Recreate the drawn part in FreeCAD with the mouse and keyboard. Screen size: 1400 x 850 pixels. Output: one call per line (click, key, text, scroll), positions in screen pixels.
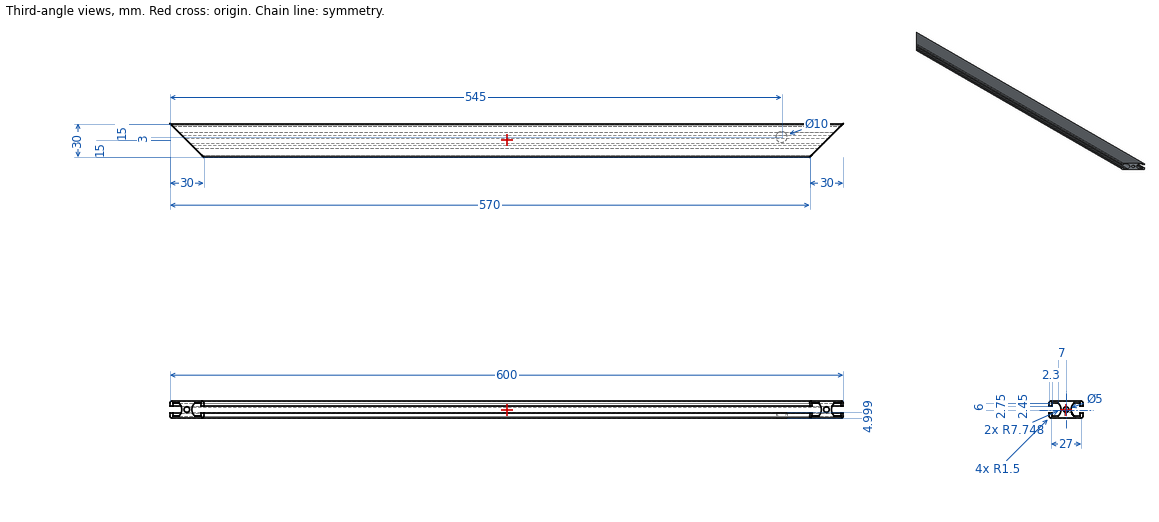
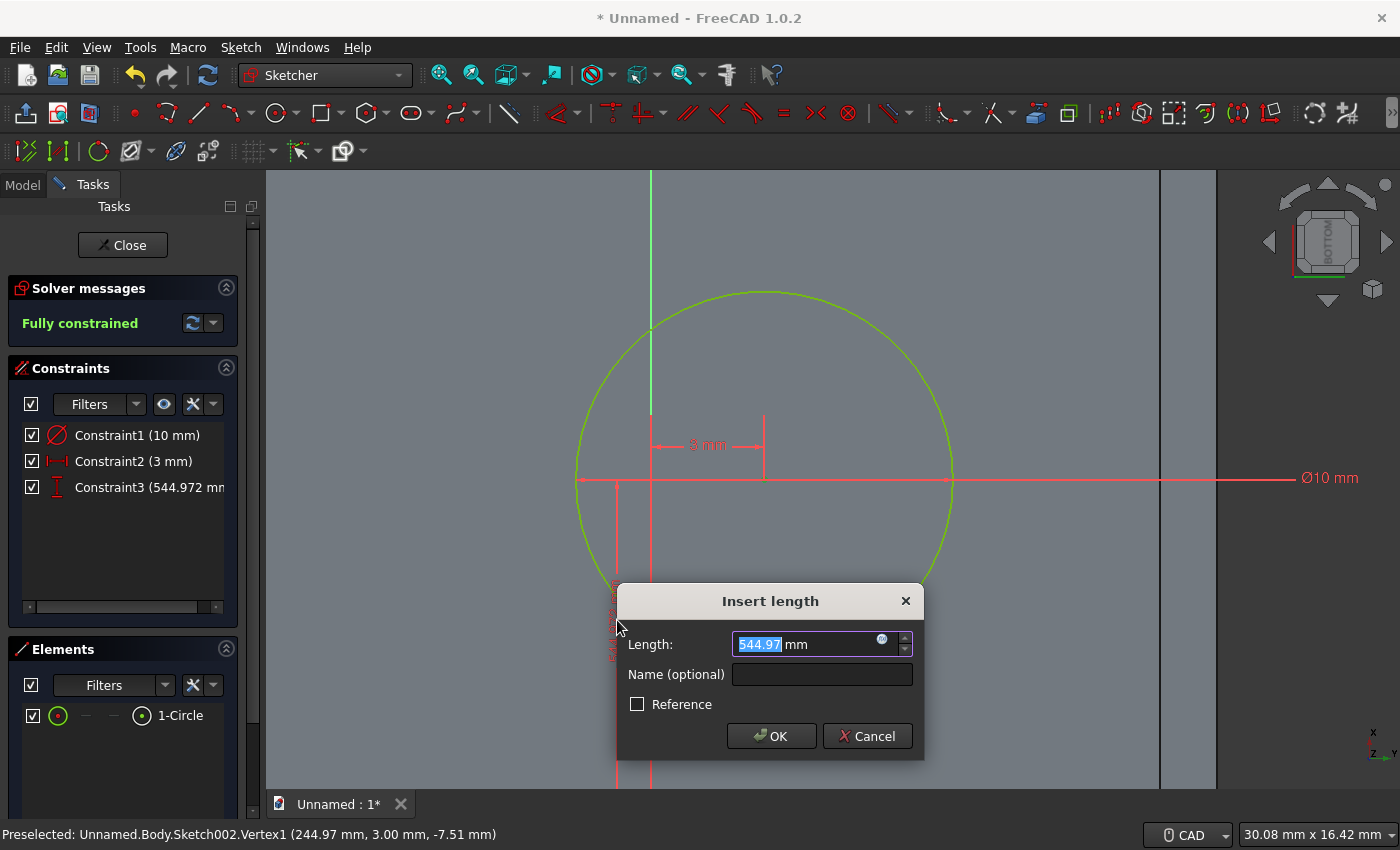
text(545)
key(Return)
key(Escape)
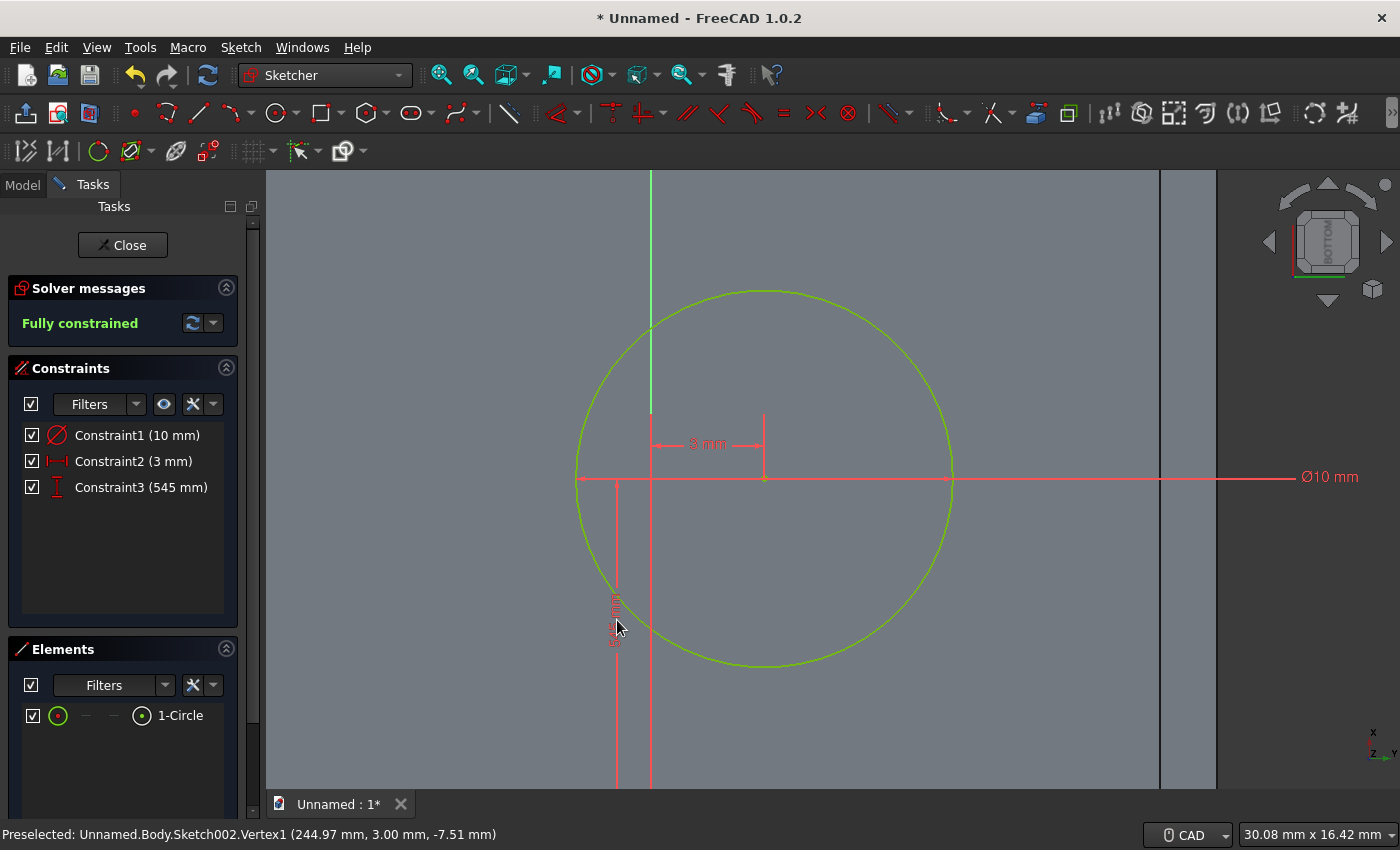
click(123, 245)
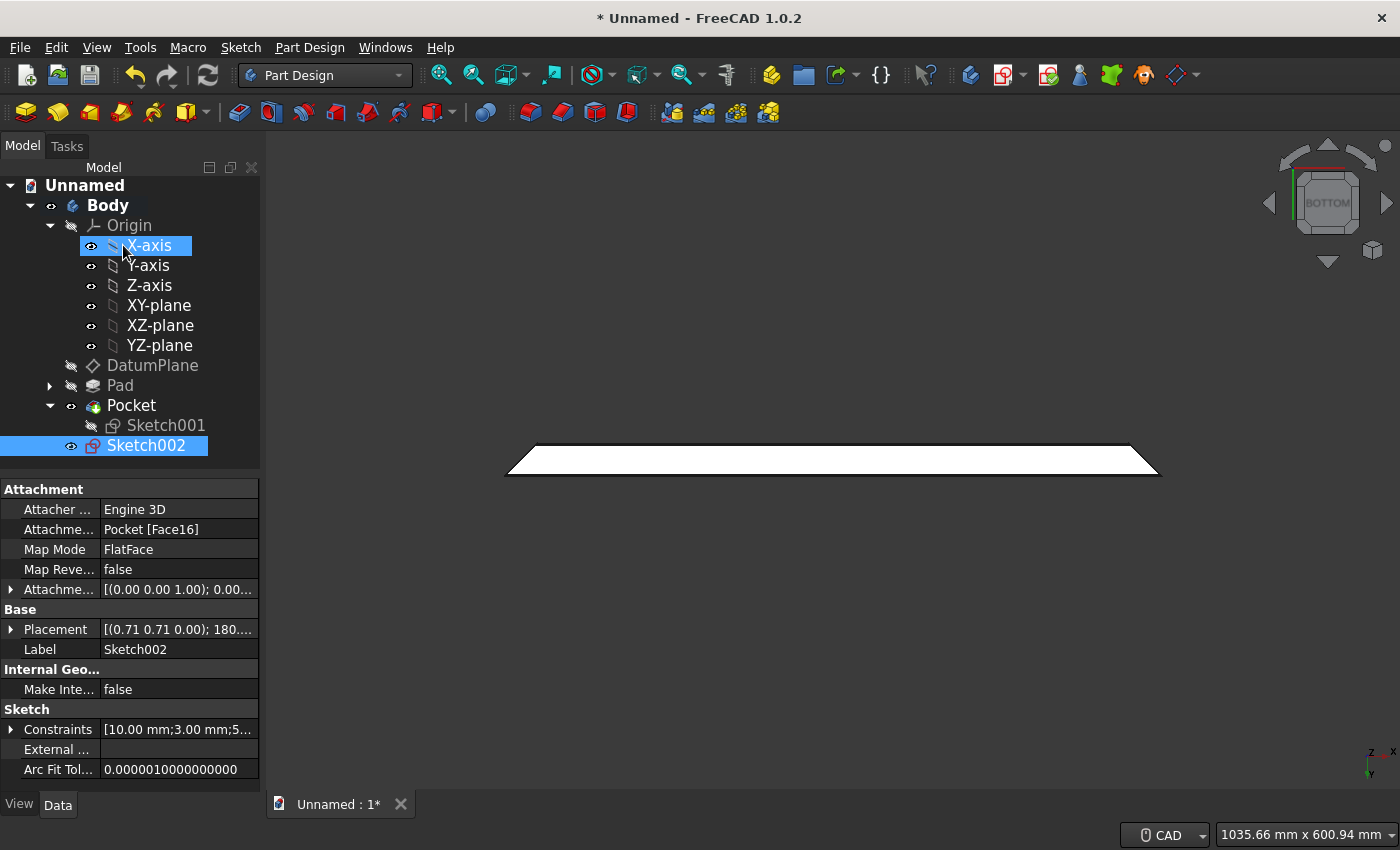
click(240, 112)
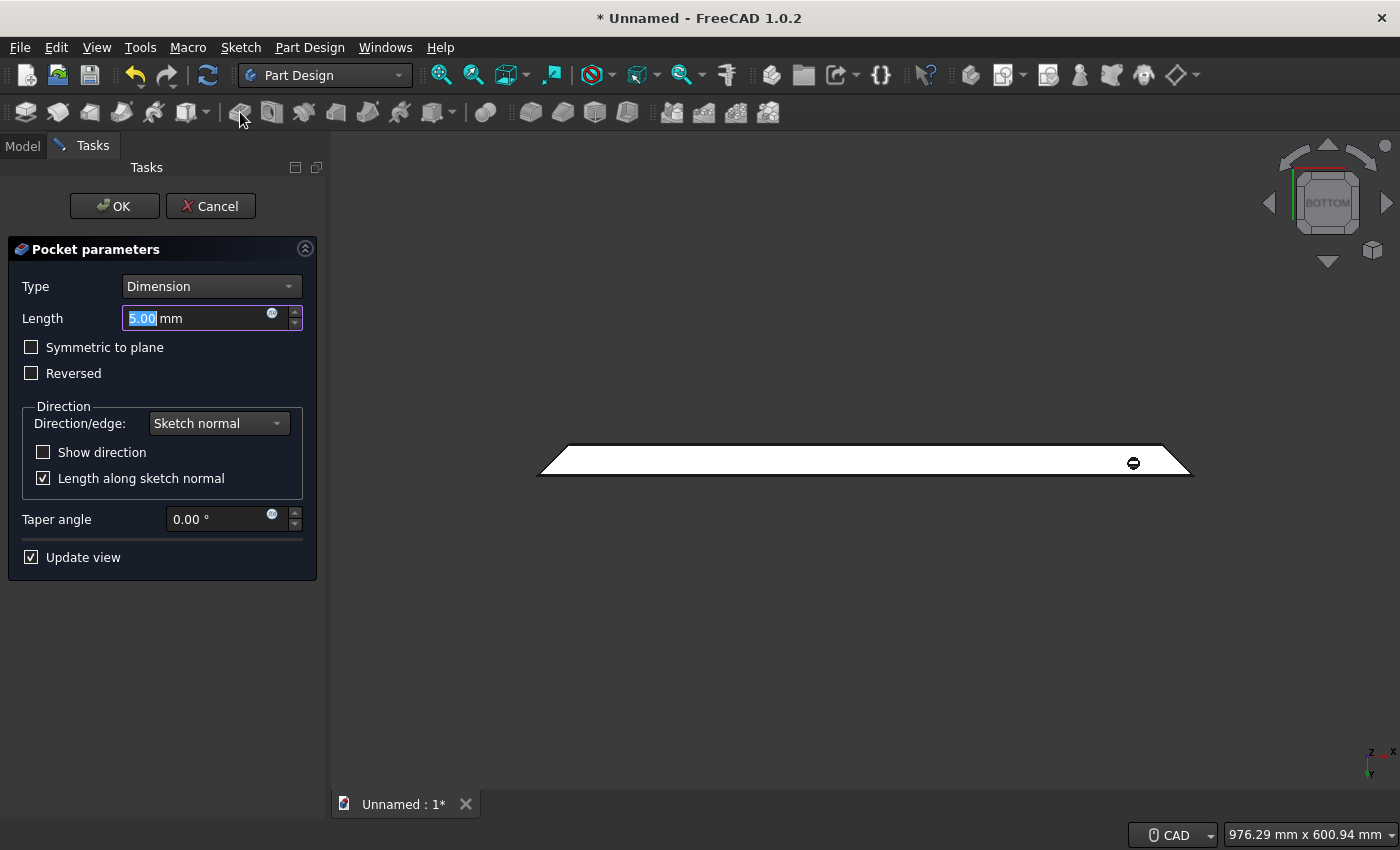
text(4.999)
key(Tab)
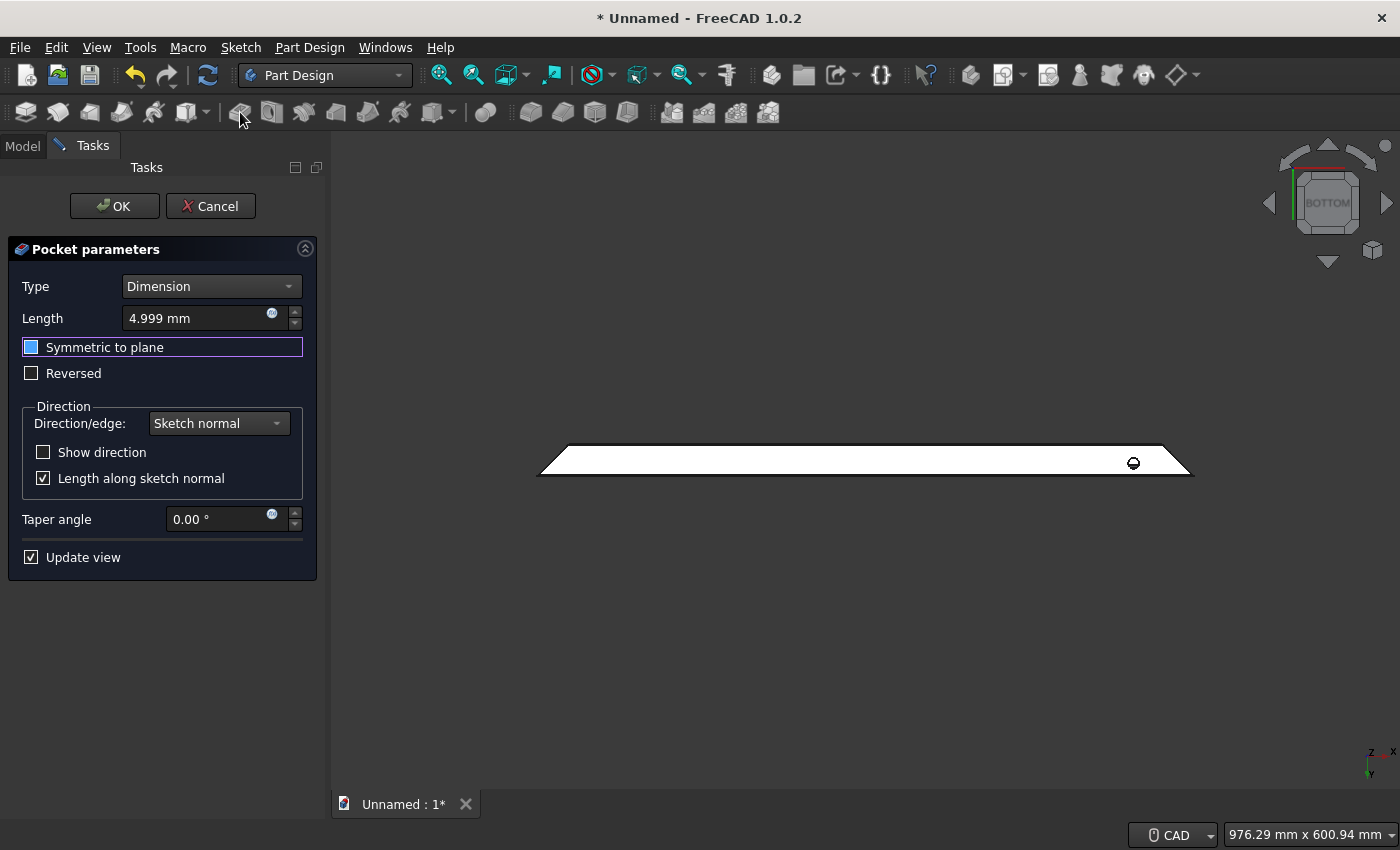
click(115, 206)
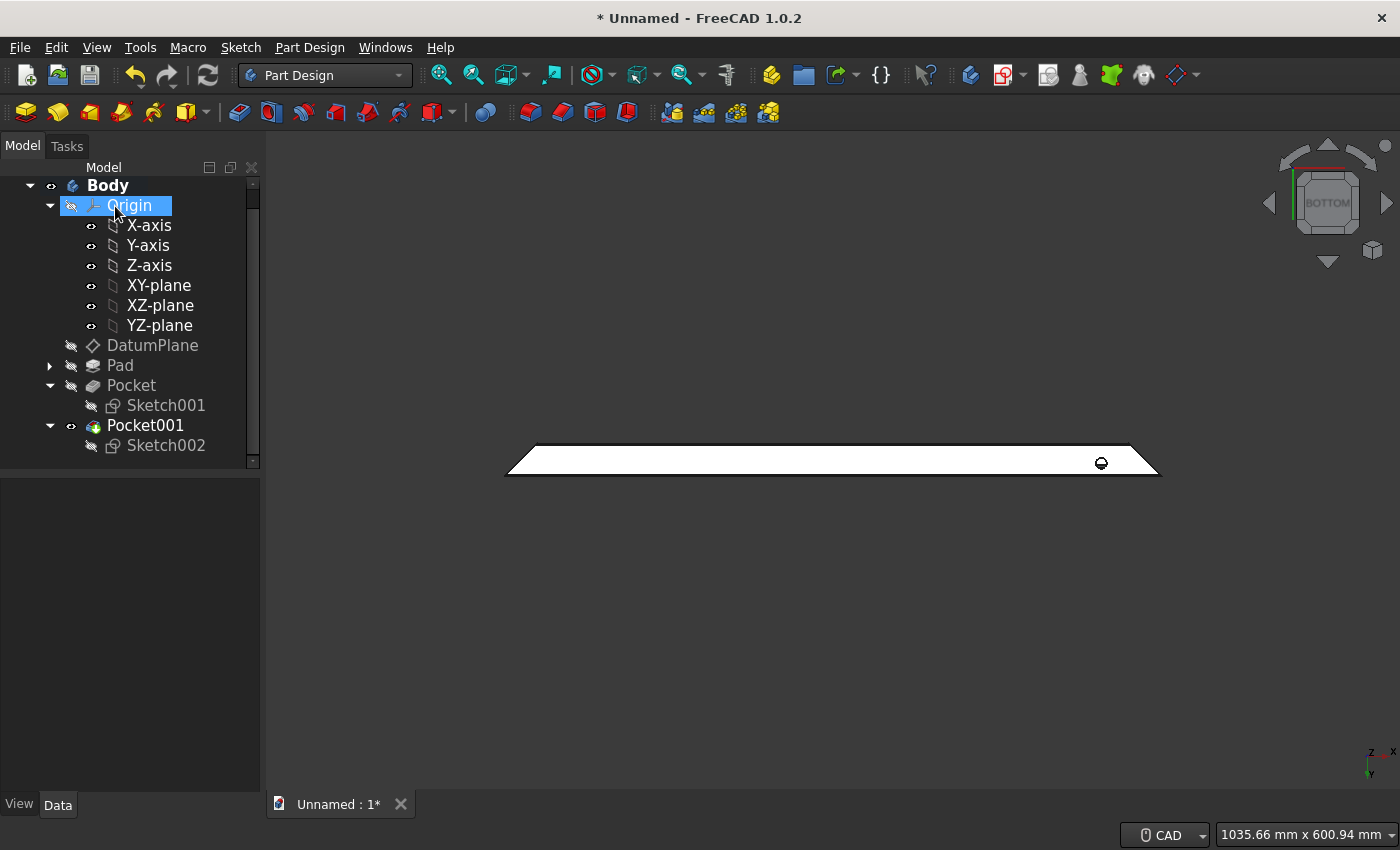
key(0)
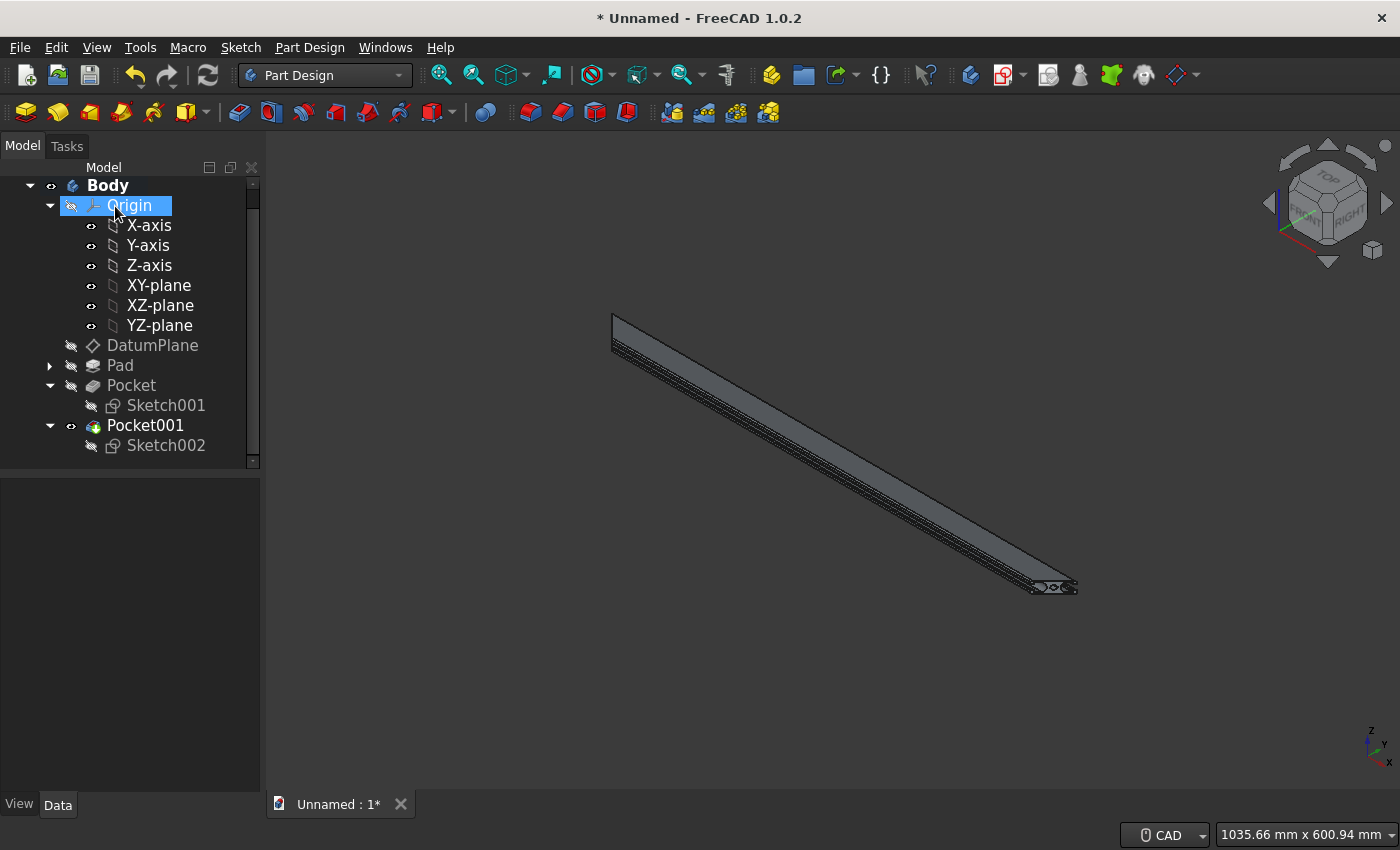
key(v)
key(f)